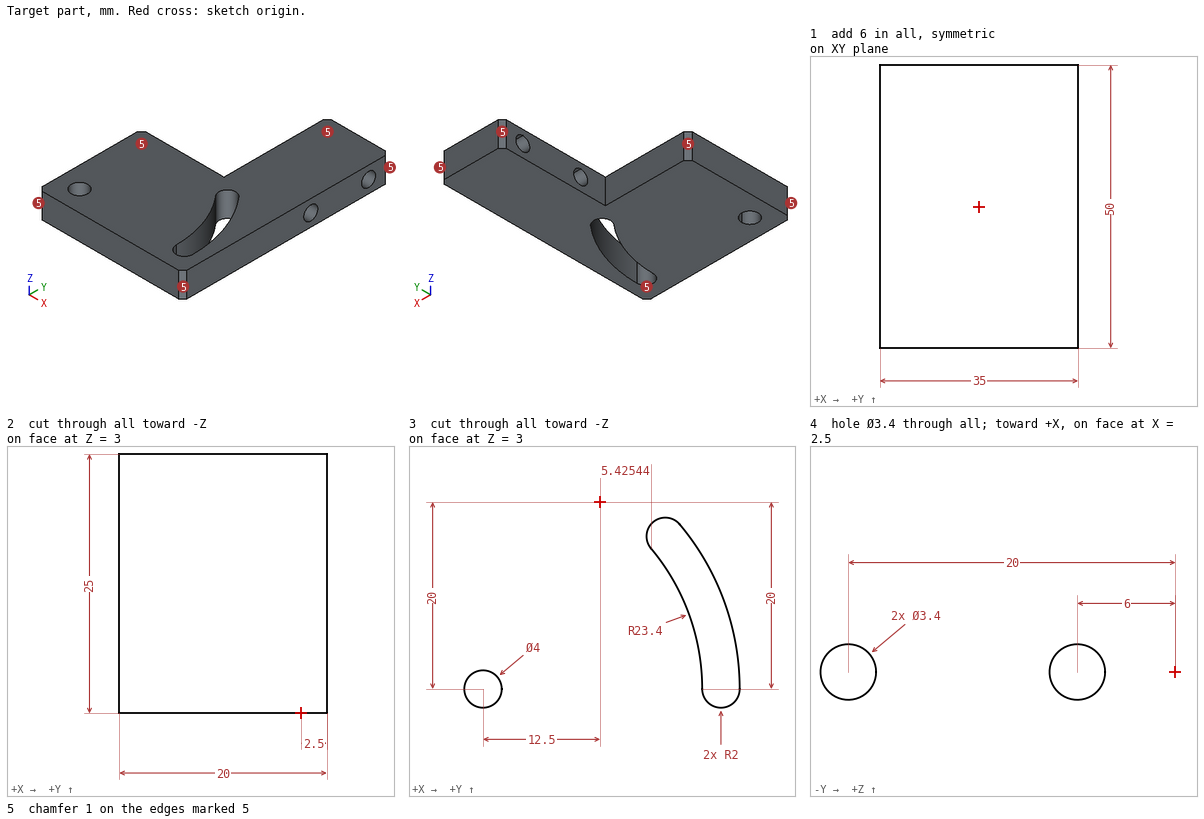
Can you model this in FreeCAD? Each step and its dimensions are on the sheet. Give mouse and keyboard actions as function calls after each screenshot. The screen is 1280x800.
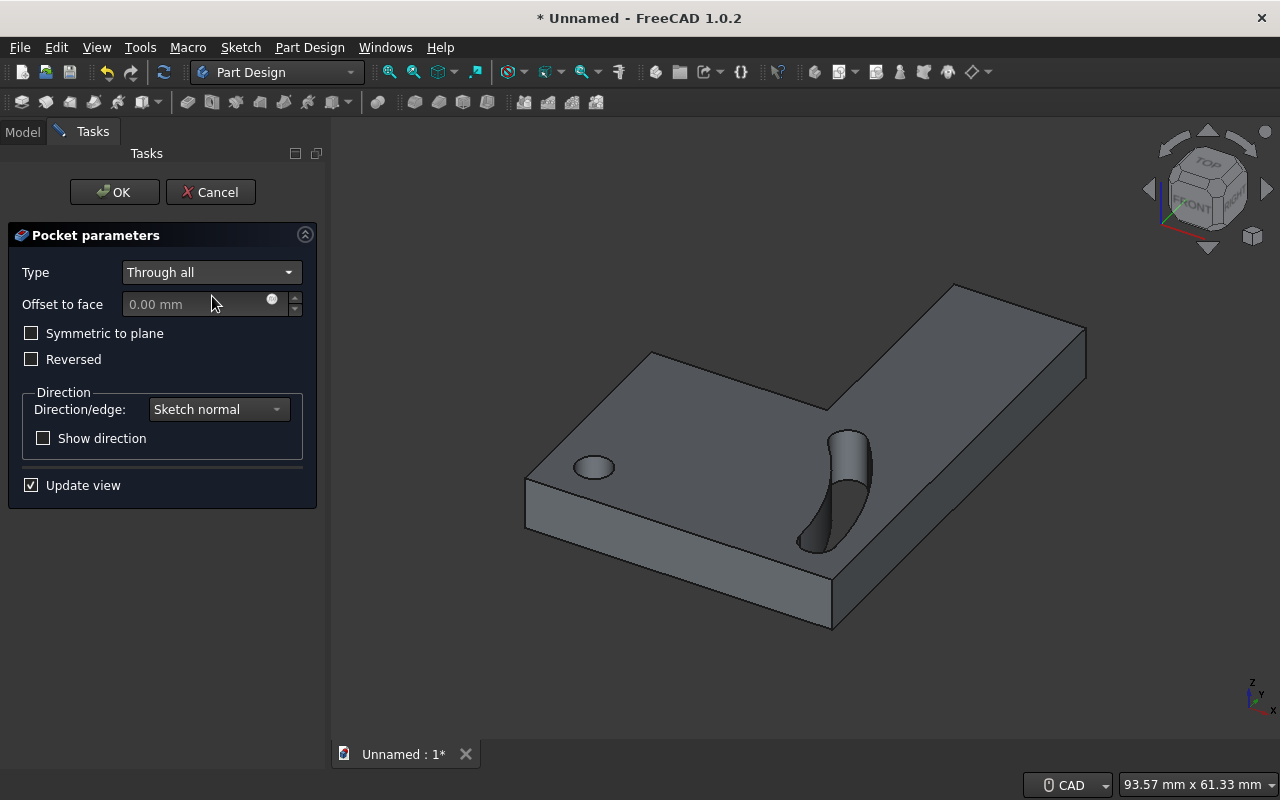
click(115, 192)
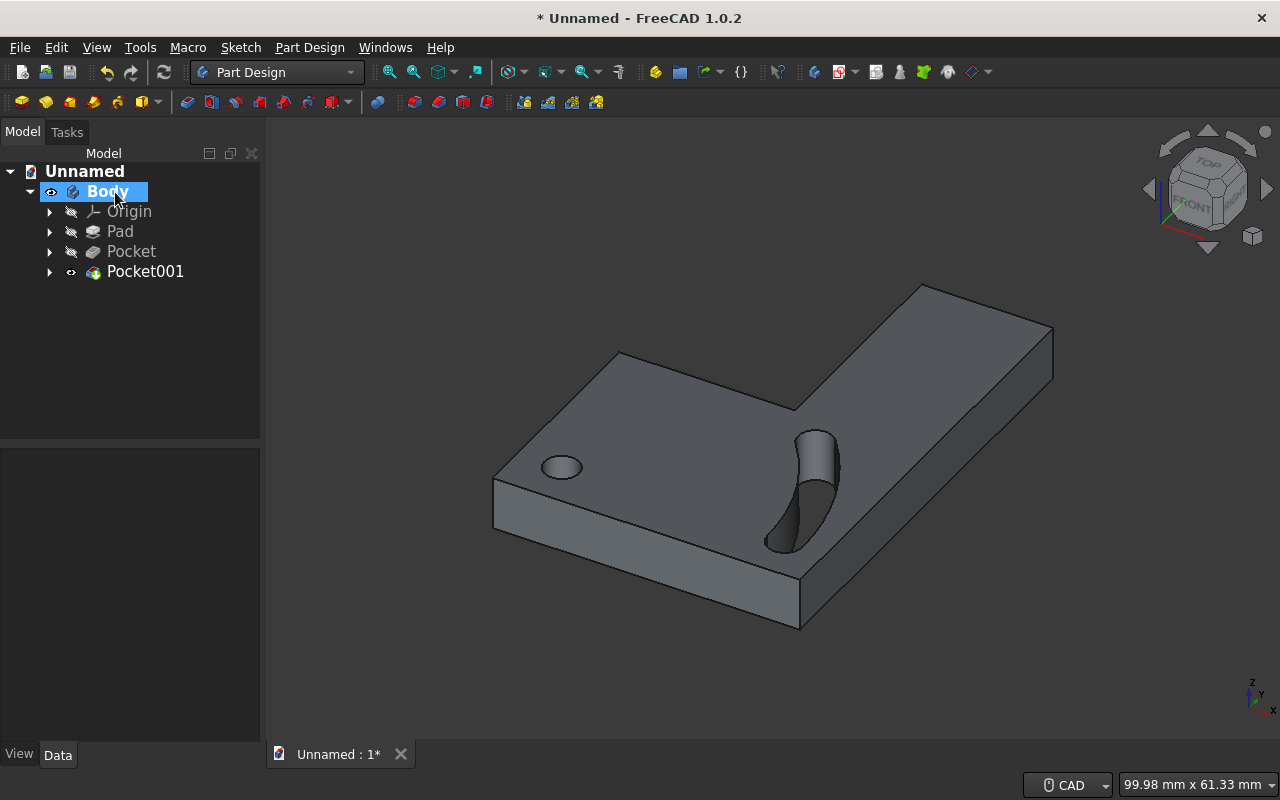
key(6)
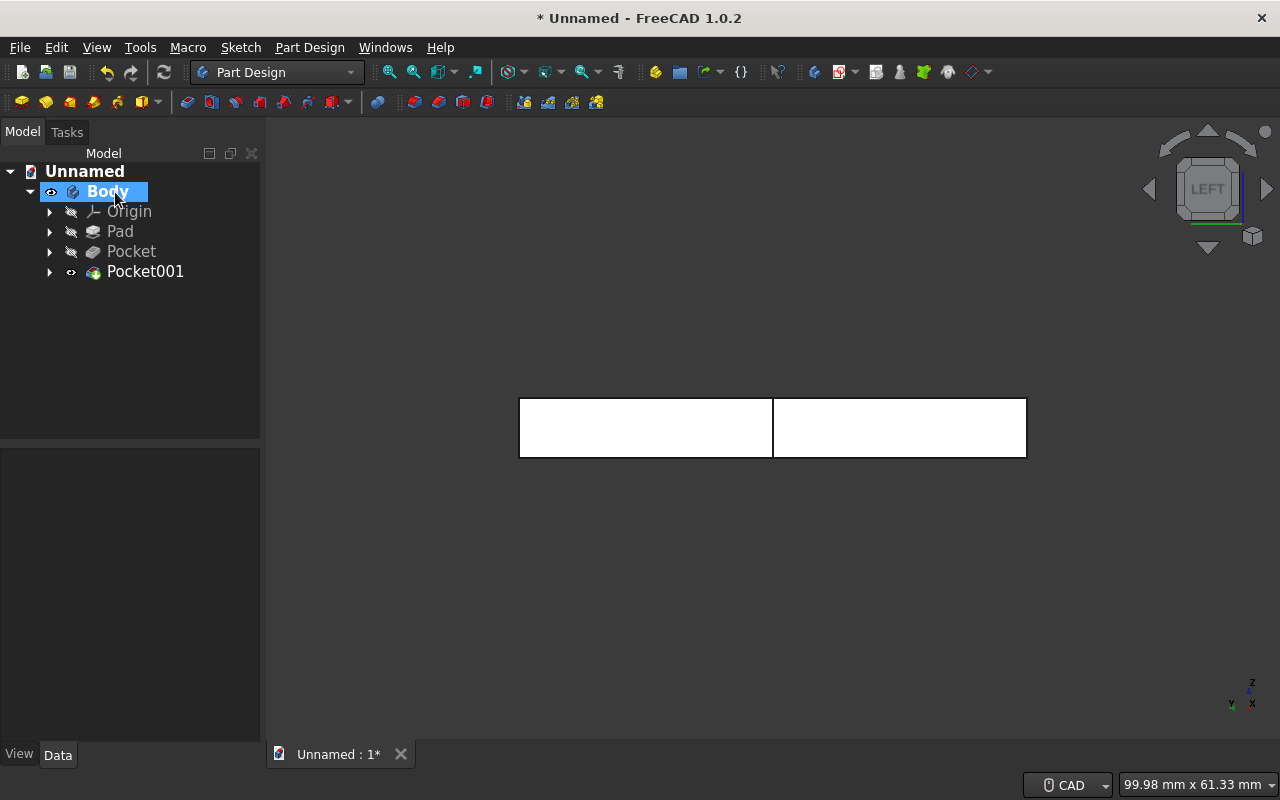
click(574, 427)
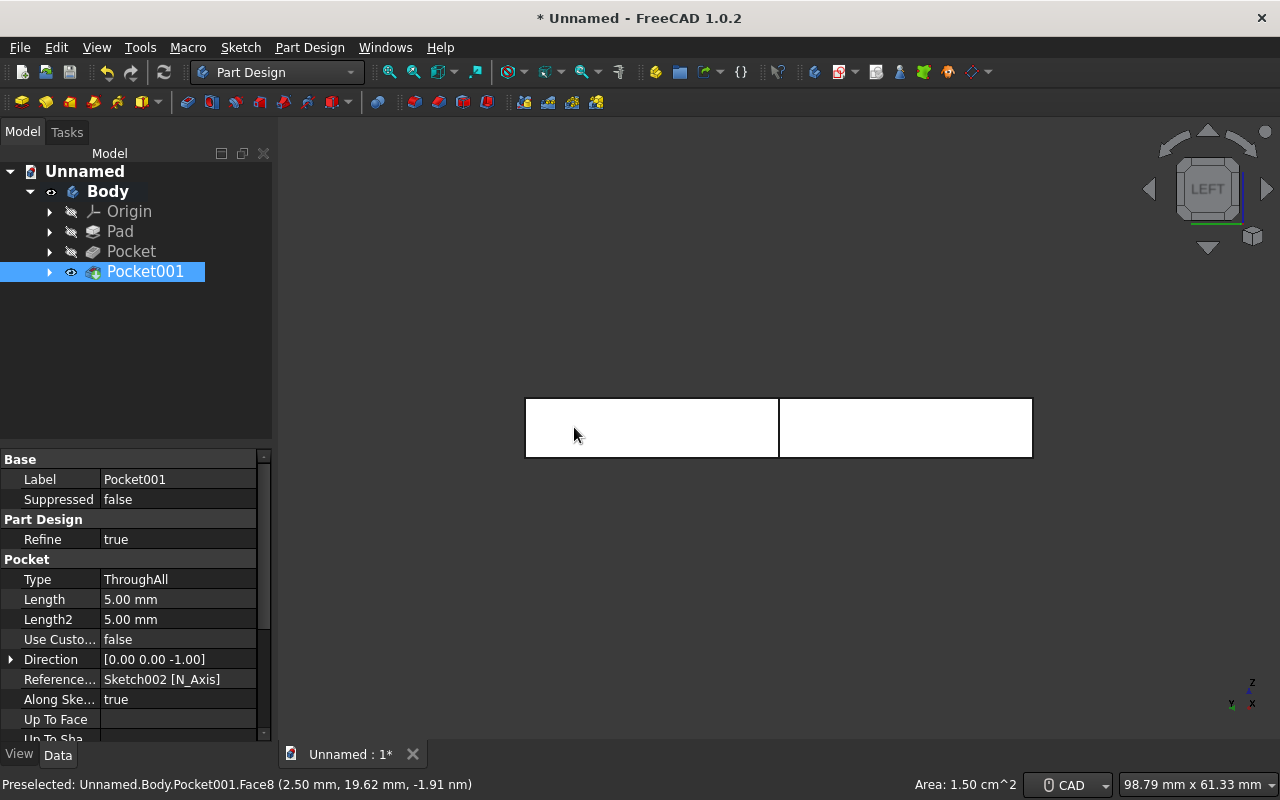
click(840, 72)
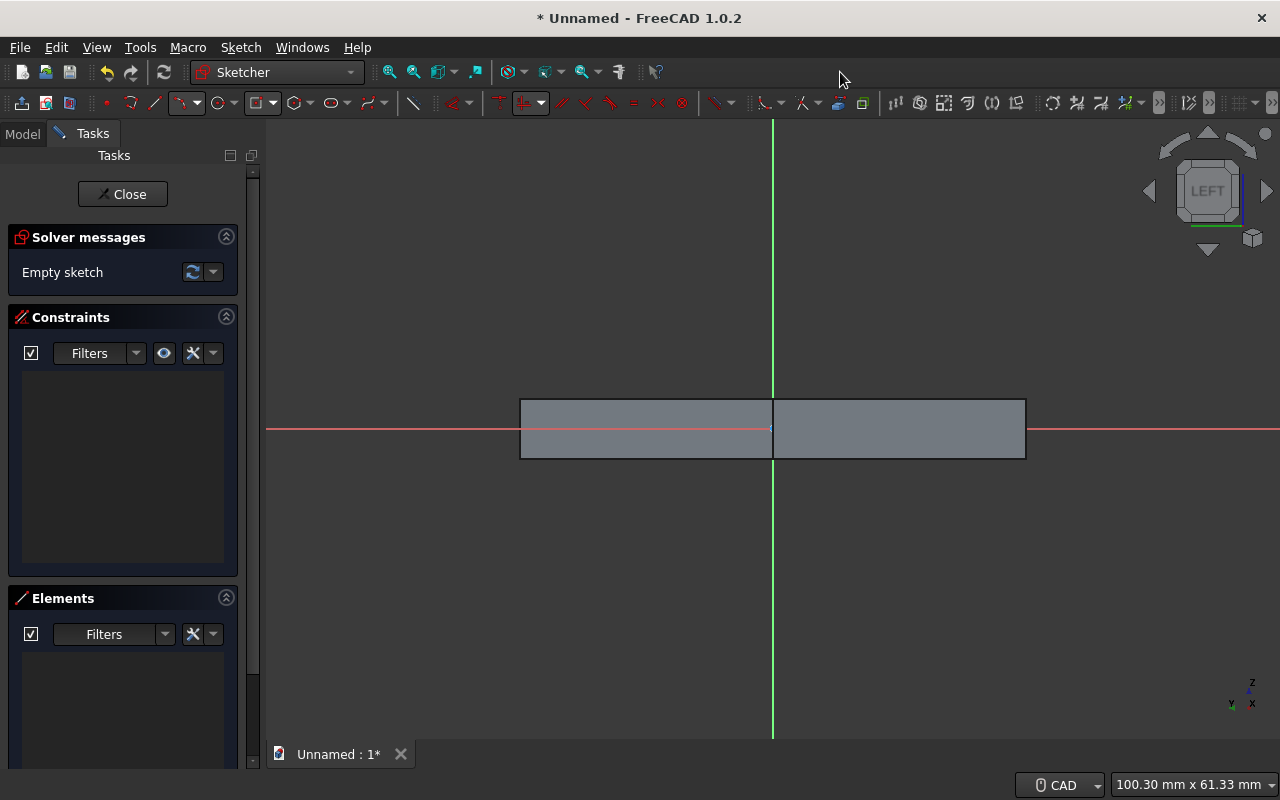
click(70, 104)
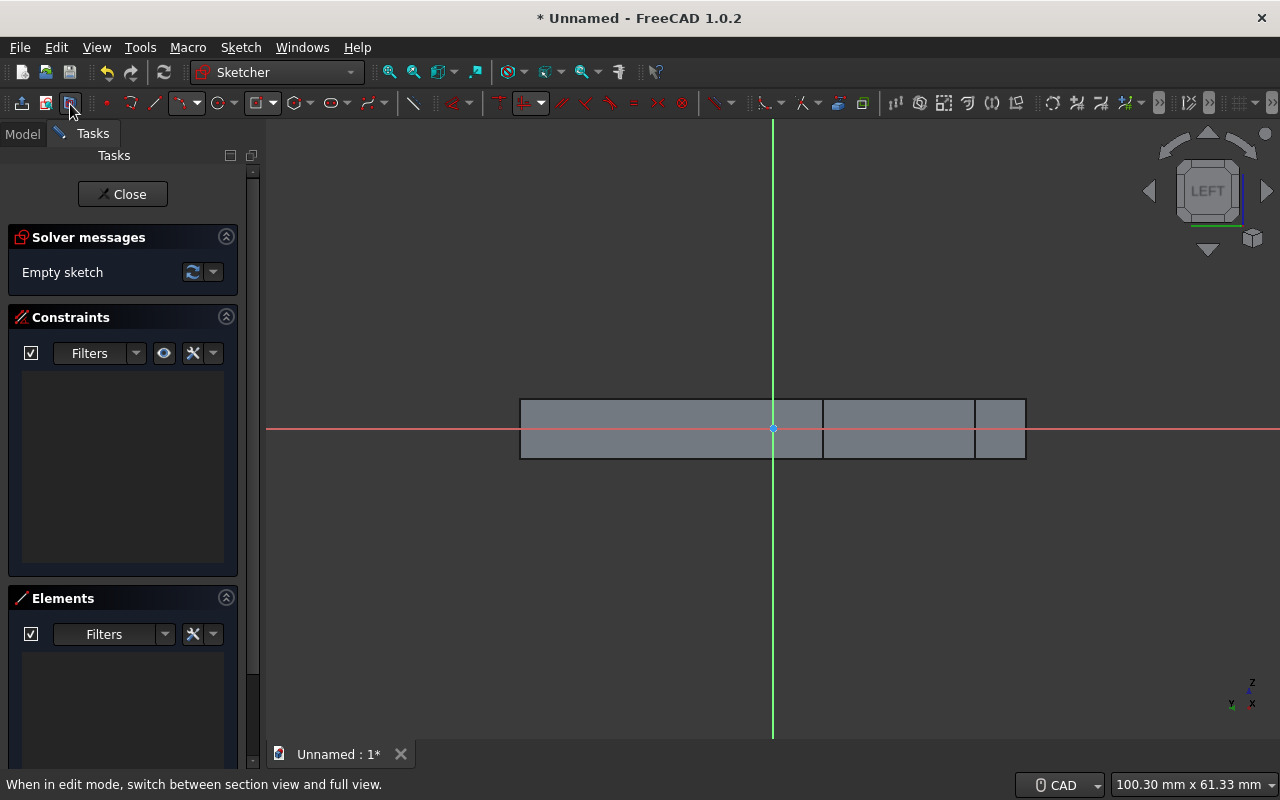
scroll(639, 429, up, 5)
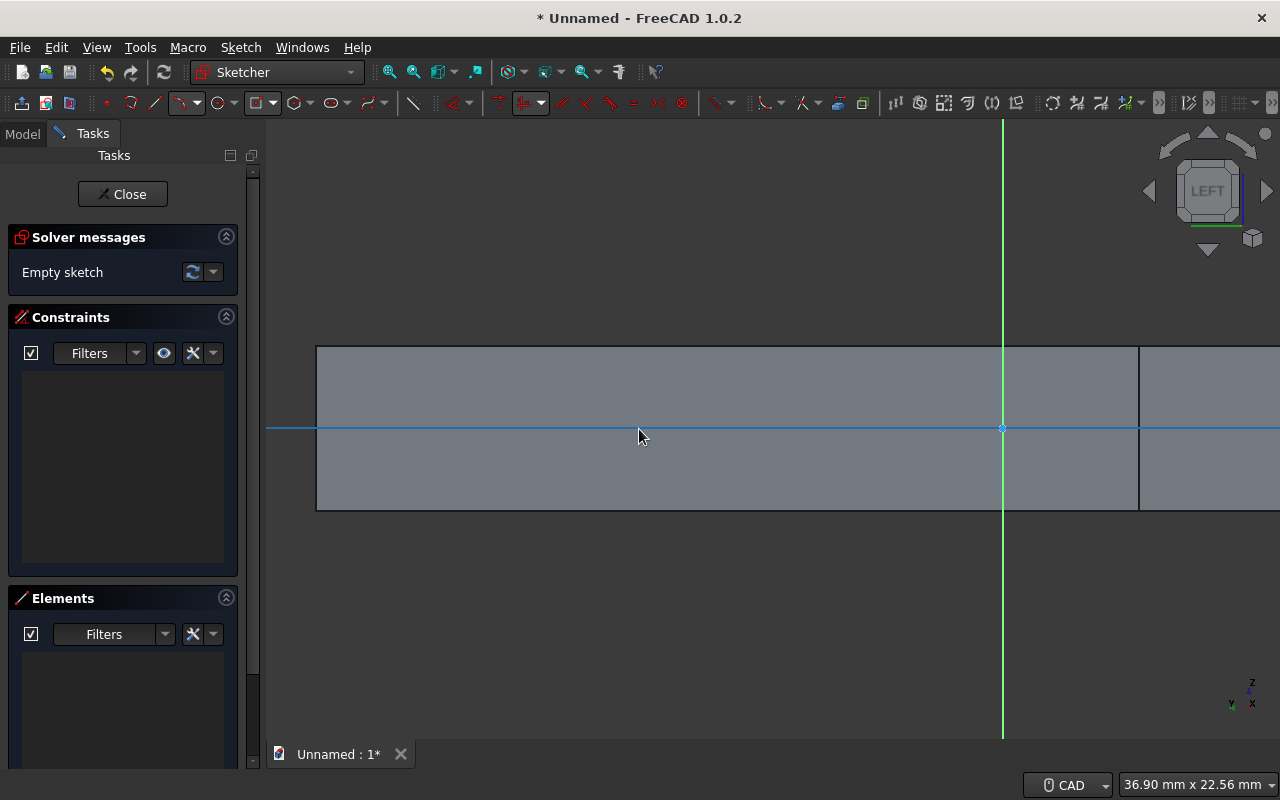
key(g)
key(c)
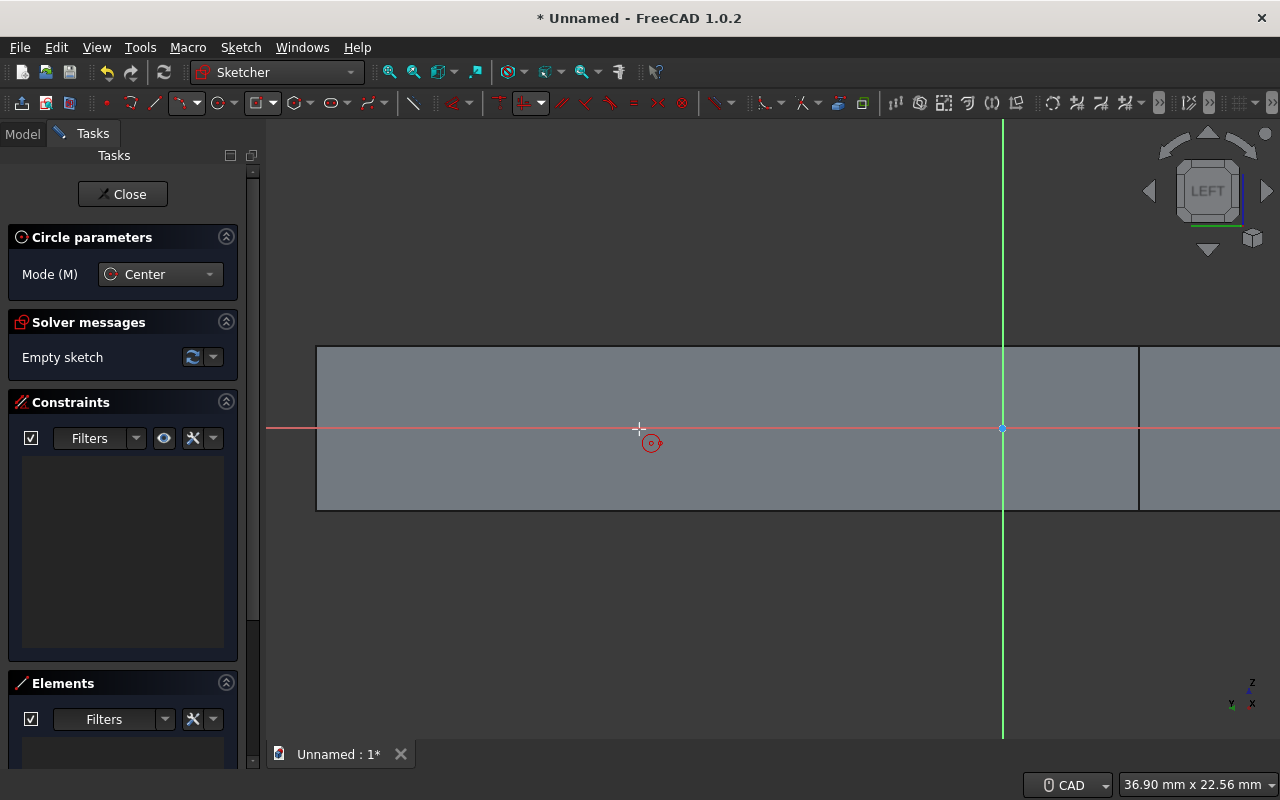
click(453, 428)
click(486, 395)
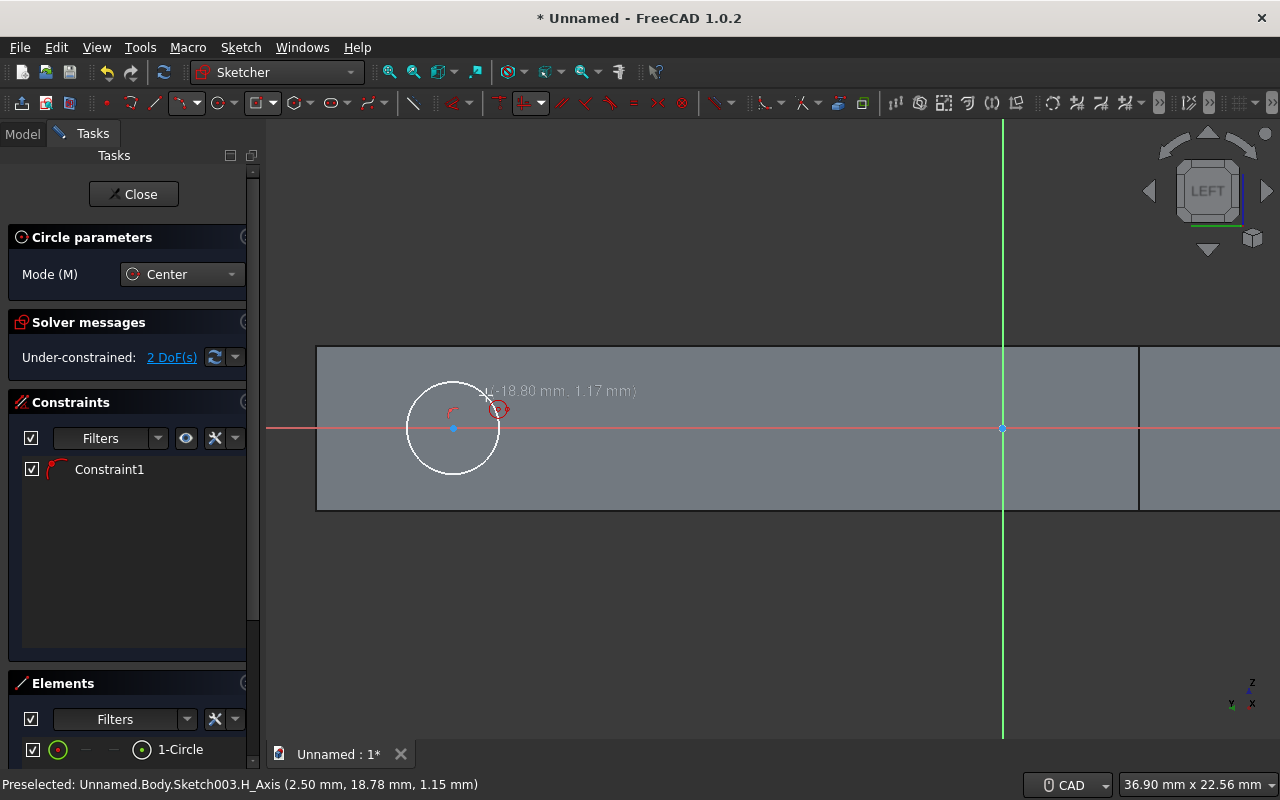
click(838, 428)
click(871, 395)
key(Escape)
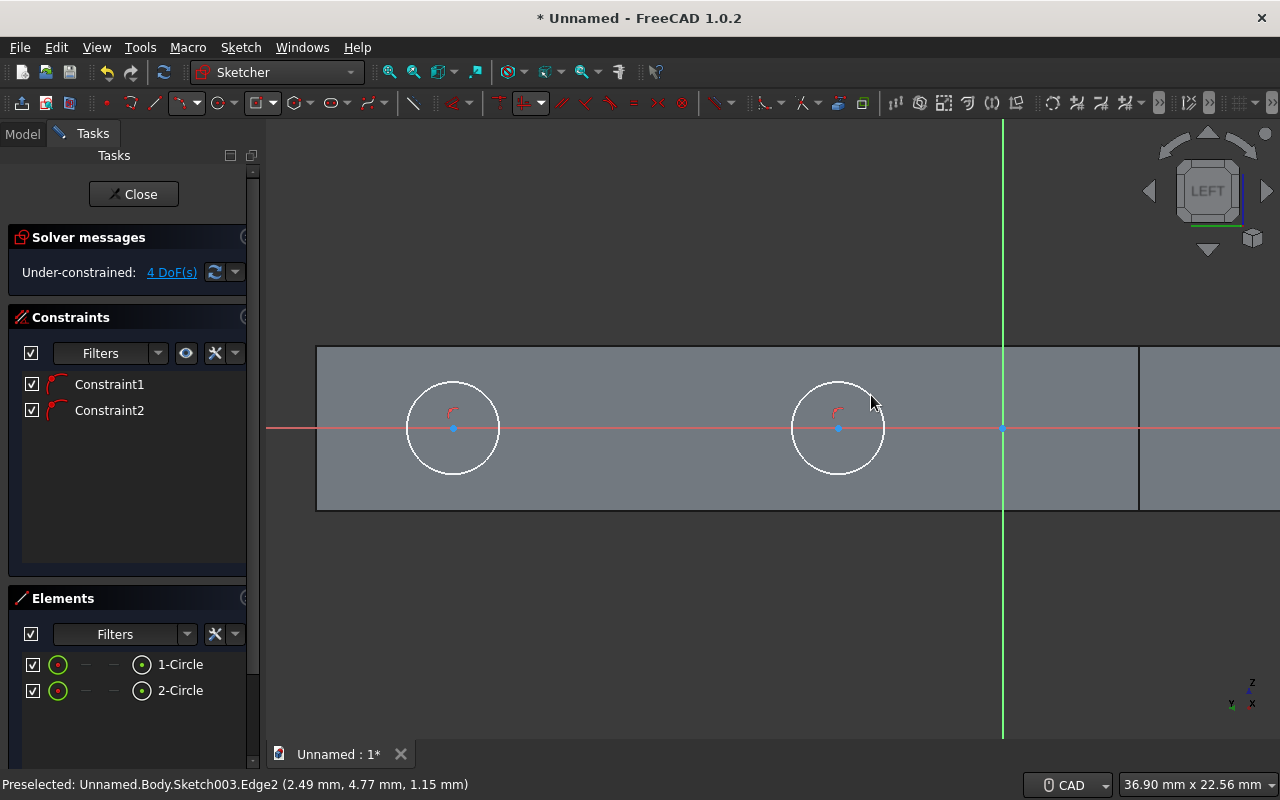
click(485, 395)